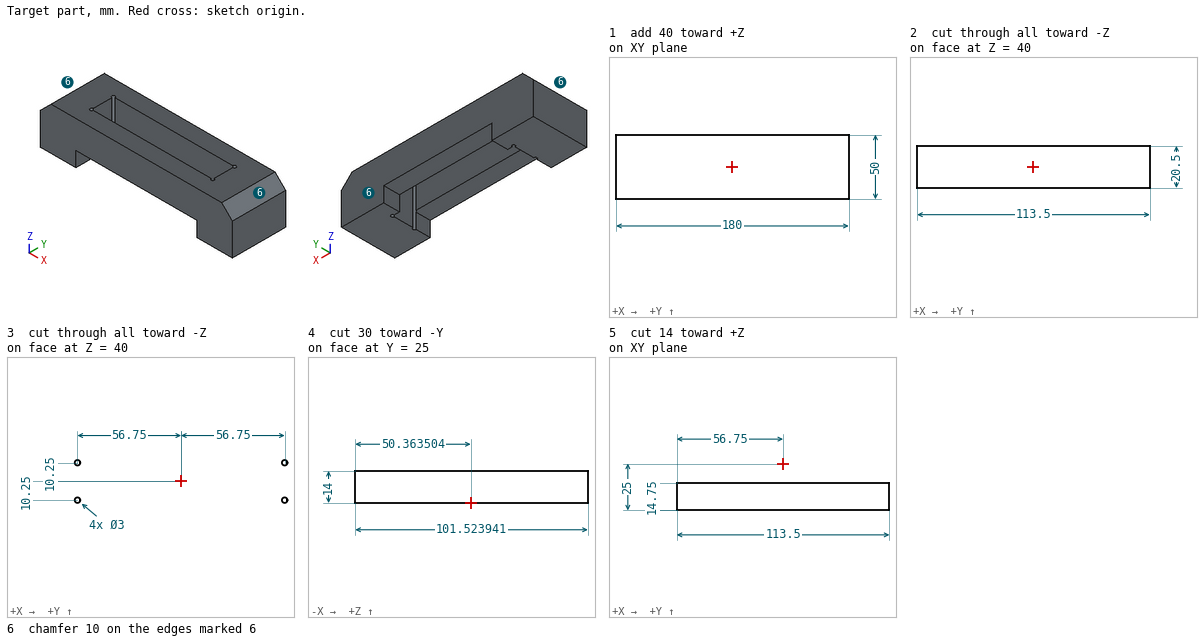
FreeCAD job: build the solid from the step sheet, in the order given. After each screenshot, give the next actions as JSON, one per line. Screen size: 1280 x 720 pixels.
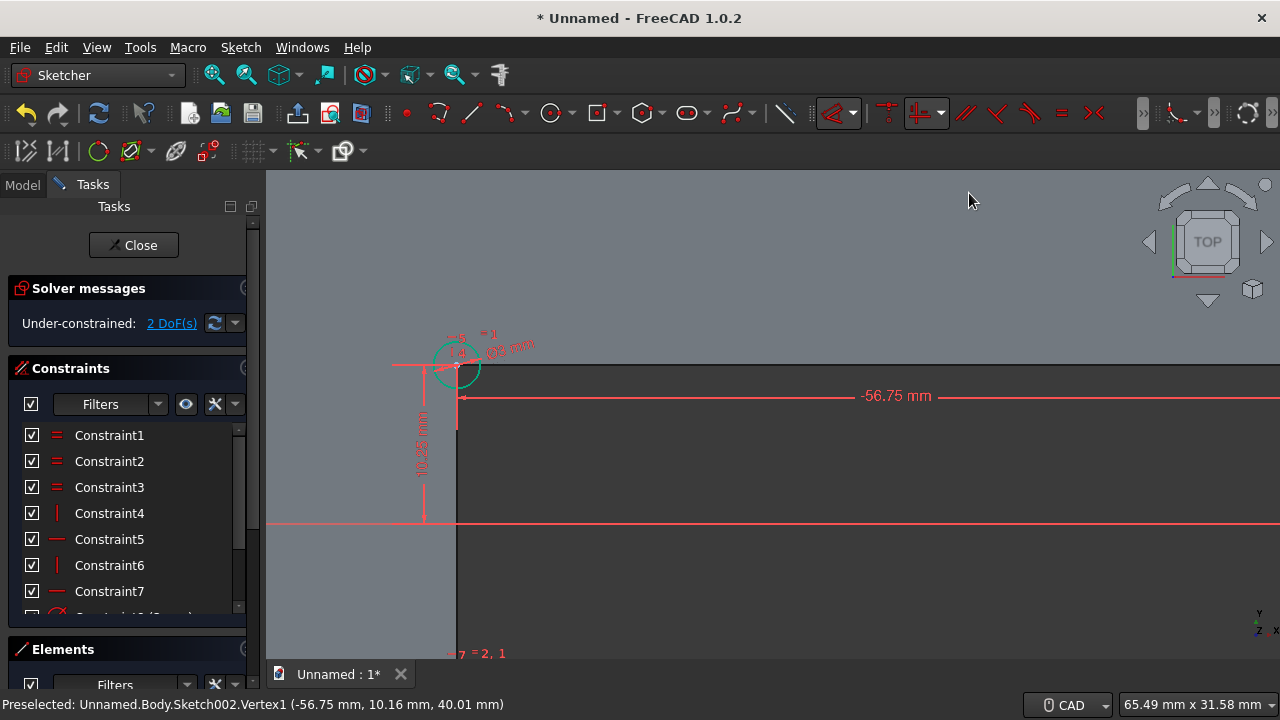
{"action": "scroll", "coordinate": [432, 367], "scroll_direction": "down", "scroll_amount": 6}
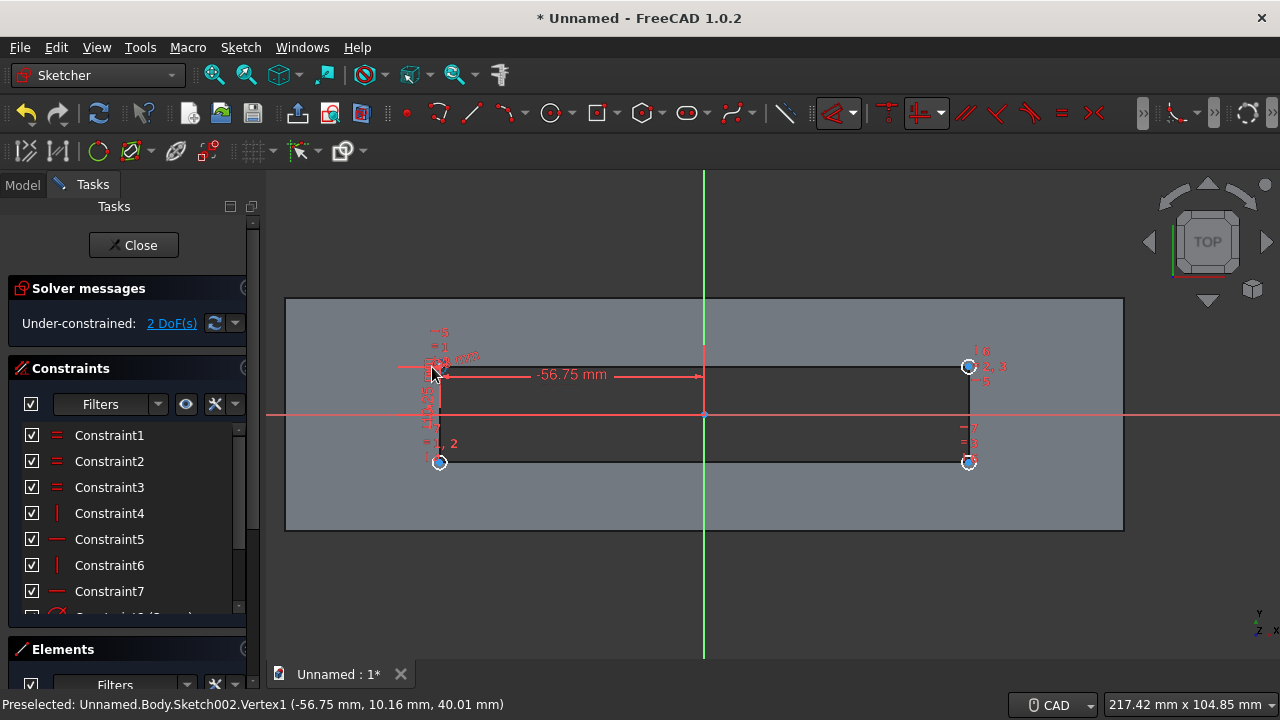
{"action": "left_click", "coordinate": [440, 463]}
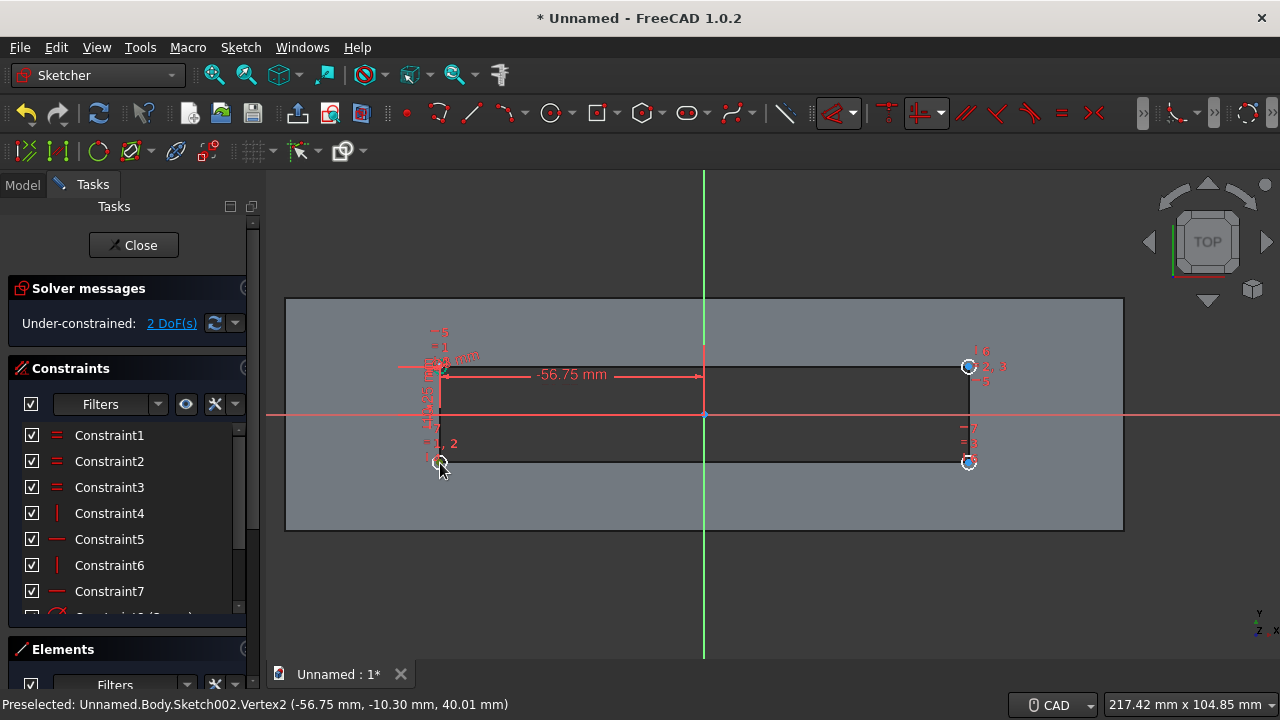
{"action": "key", "text": "i"}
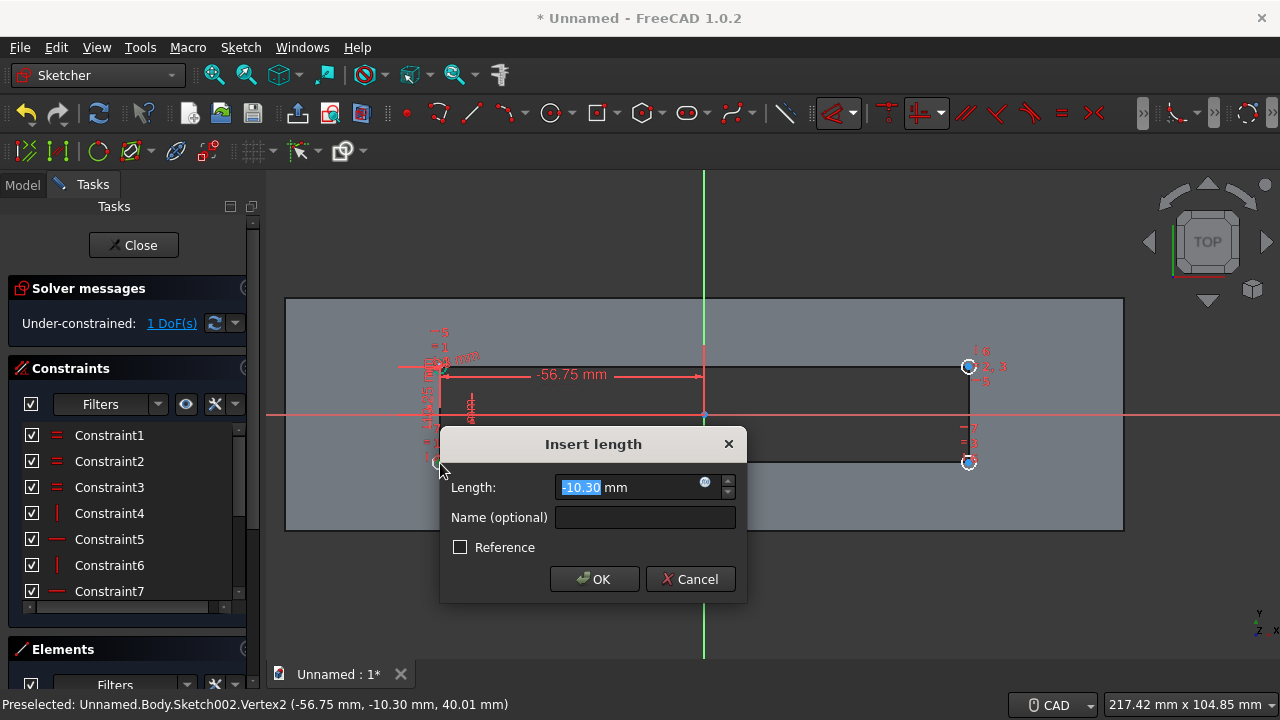
{"action": "type", "text": "-10.25"}
{"action": "key", "text": "Return"}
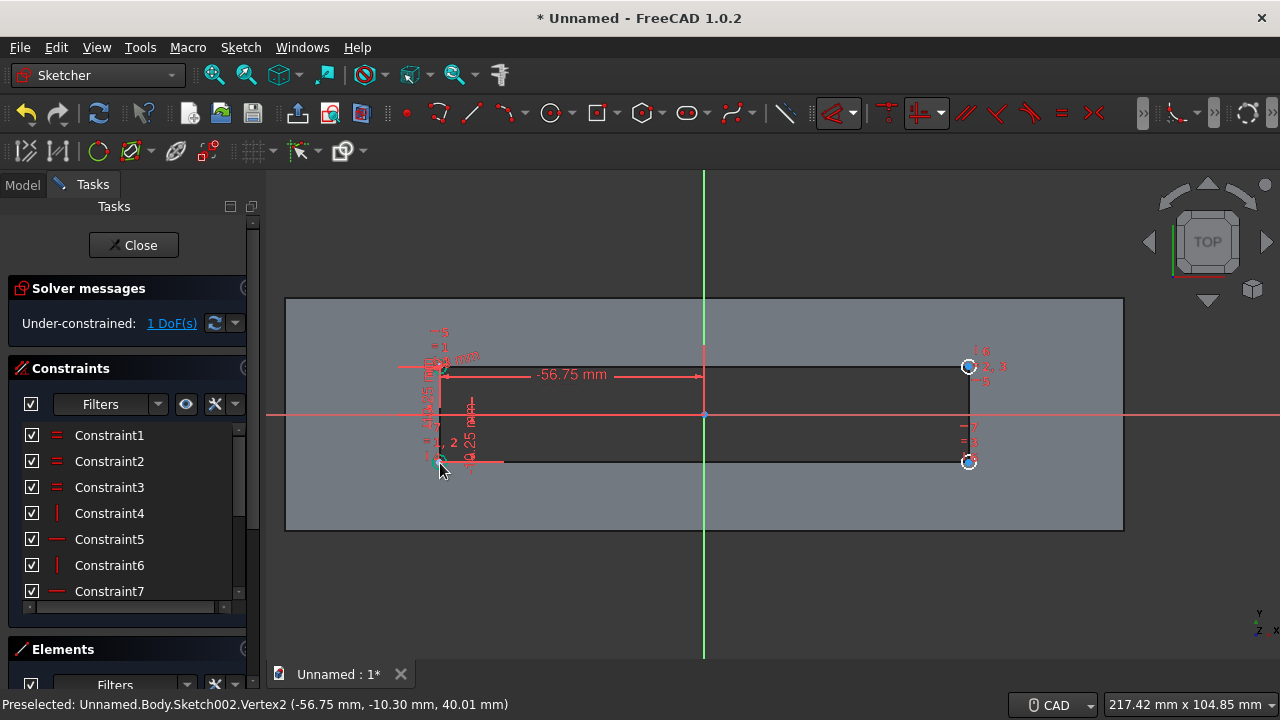
{"action": "left_click", "coordinate": [969, 367]}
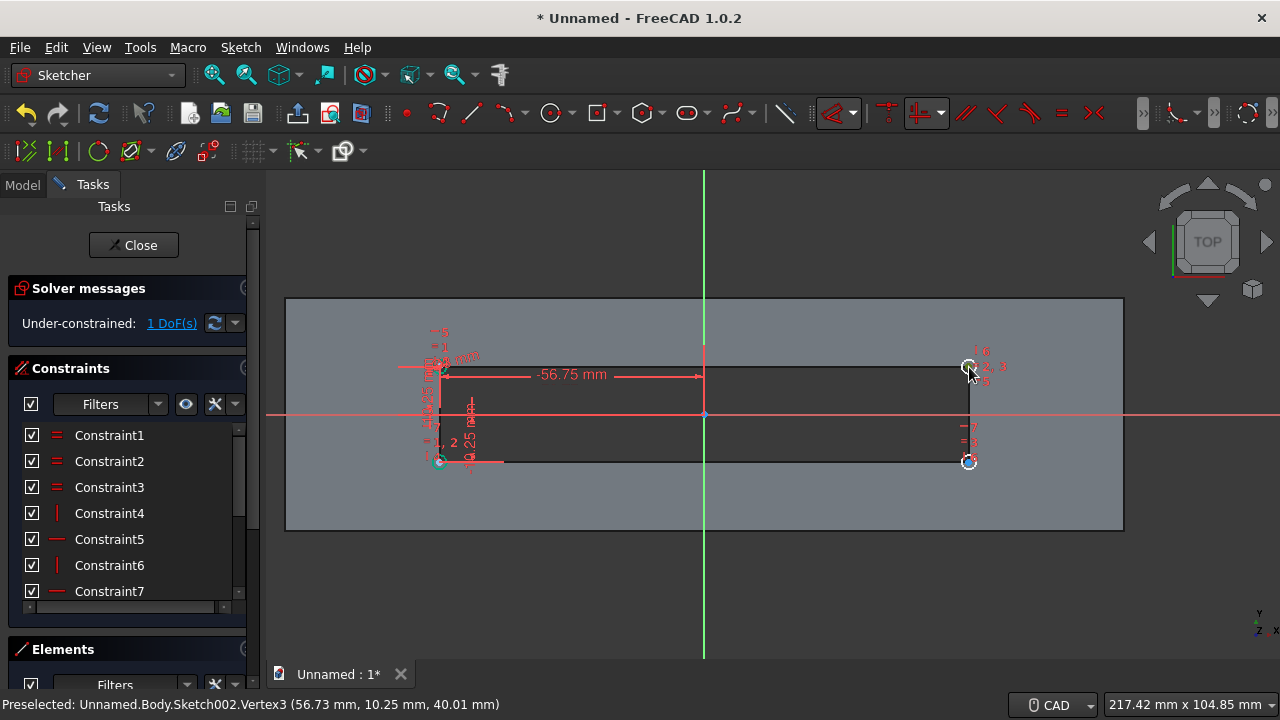
{"action": "key", "text": "l"}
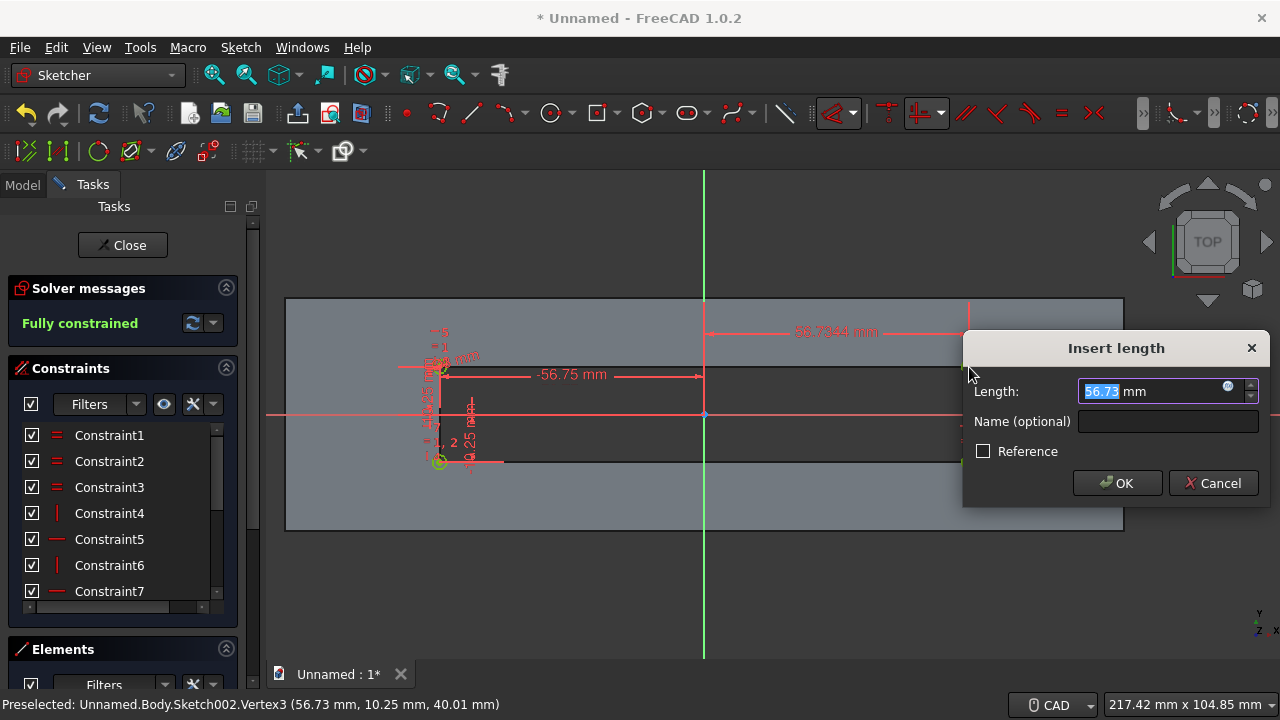
{"action": "type", "text": "56.75"}
{"action": "key", "text": "Return"}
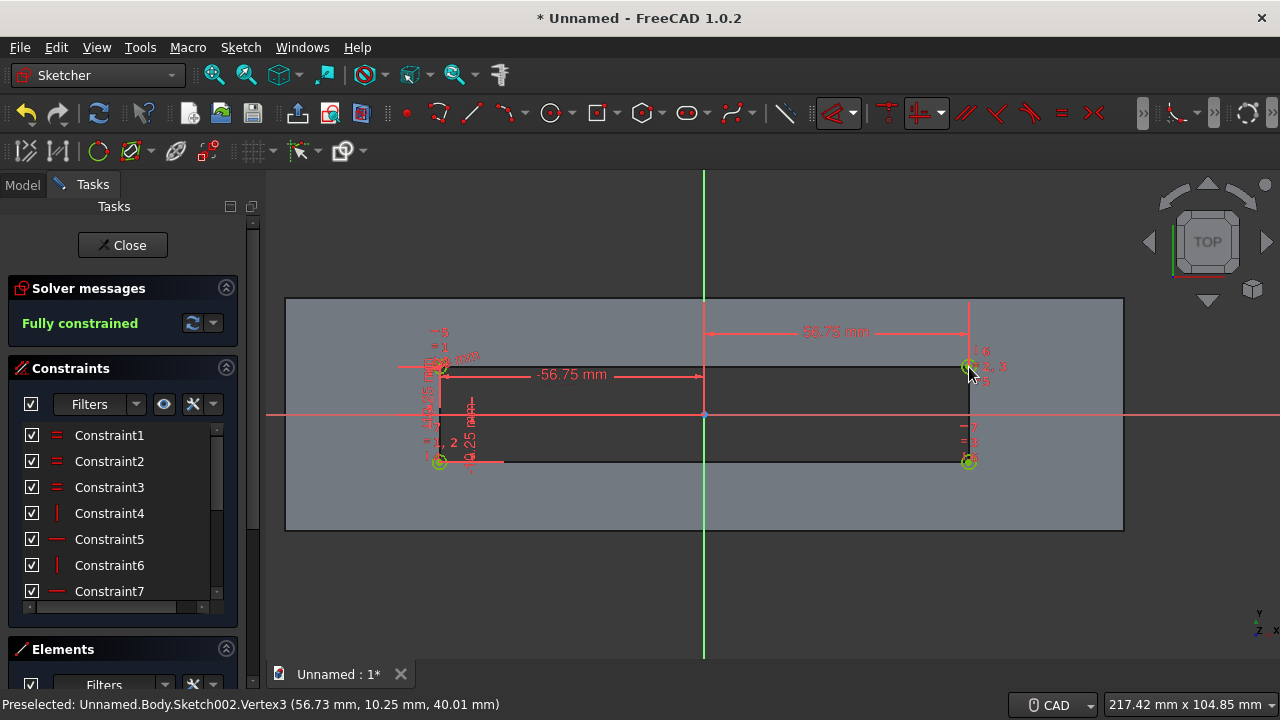
{"action": "left_click", "coordinate": [123, 245]}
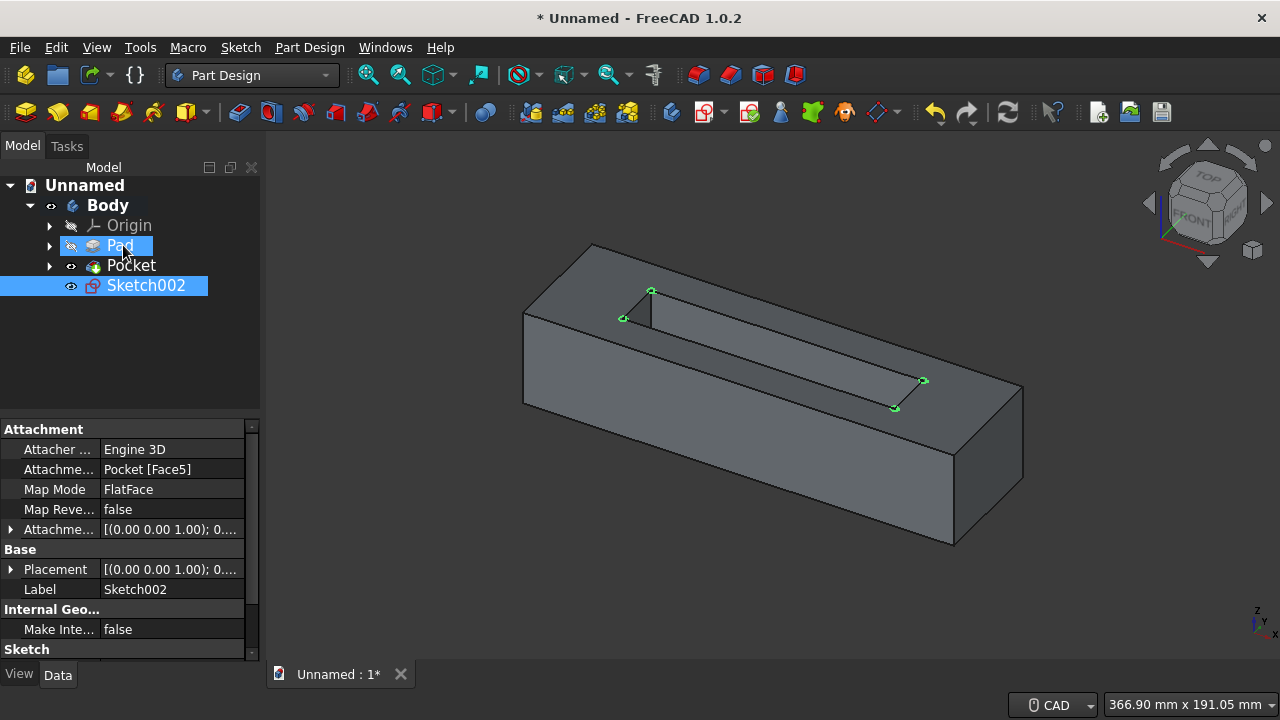
{"action": "left_click", "coordinate": [240, 112]}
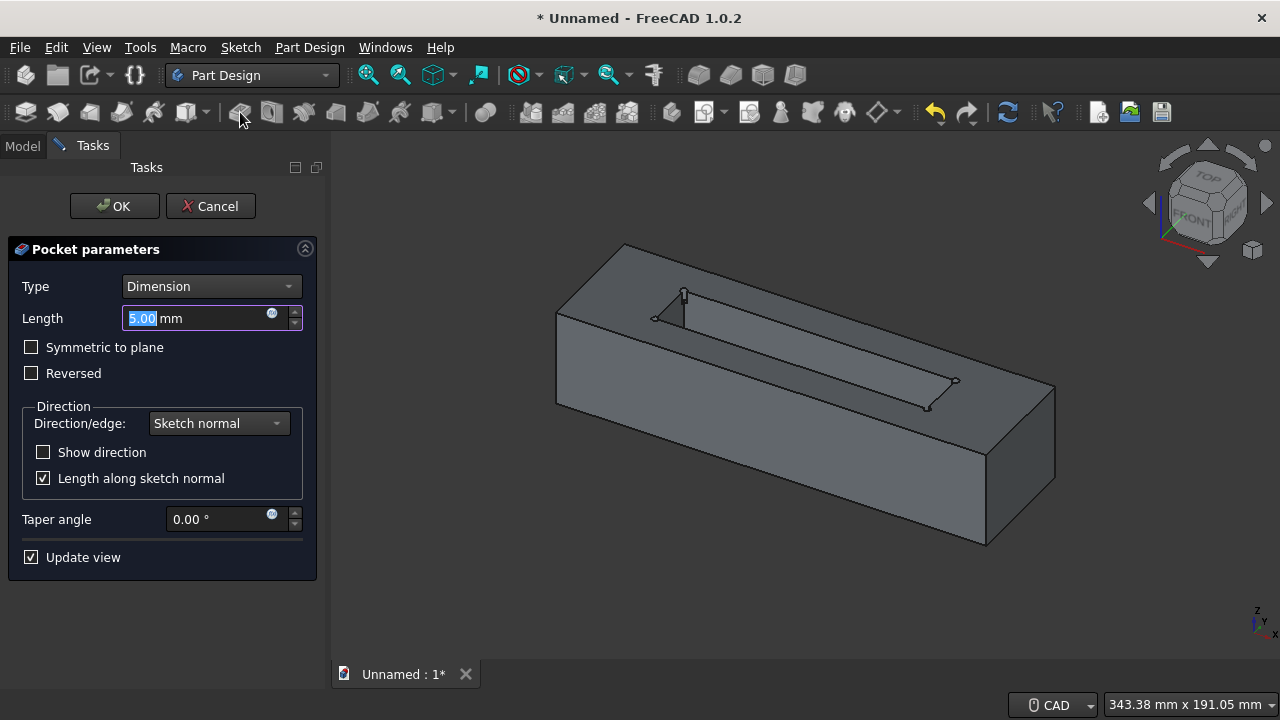
{"action": "left_click", "coordinate": [212, 286]}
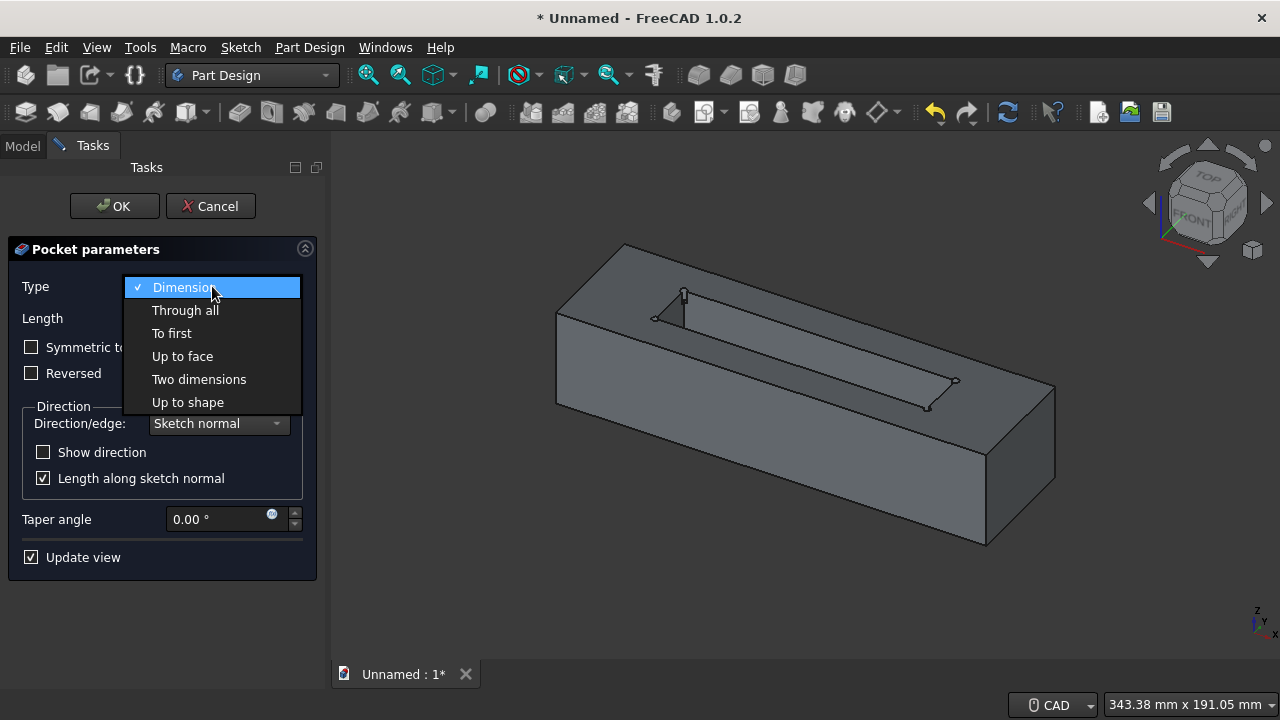
{"action": "left_click", "coordinate": [212, 310]}